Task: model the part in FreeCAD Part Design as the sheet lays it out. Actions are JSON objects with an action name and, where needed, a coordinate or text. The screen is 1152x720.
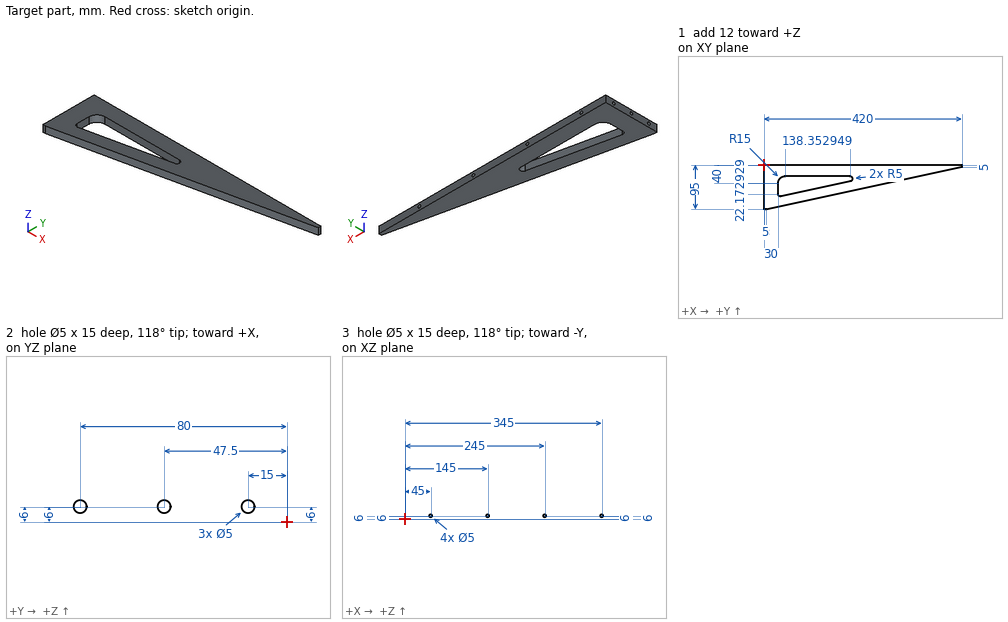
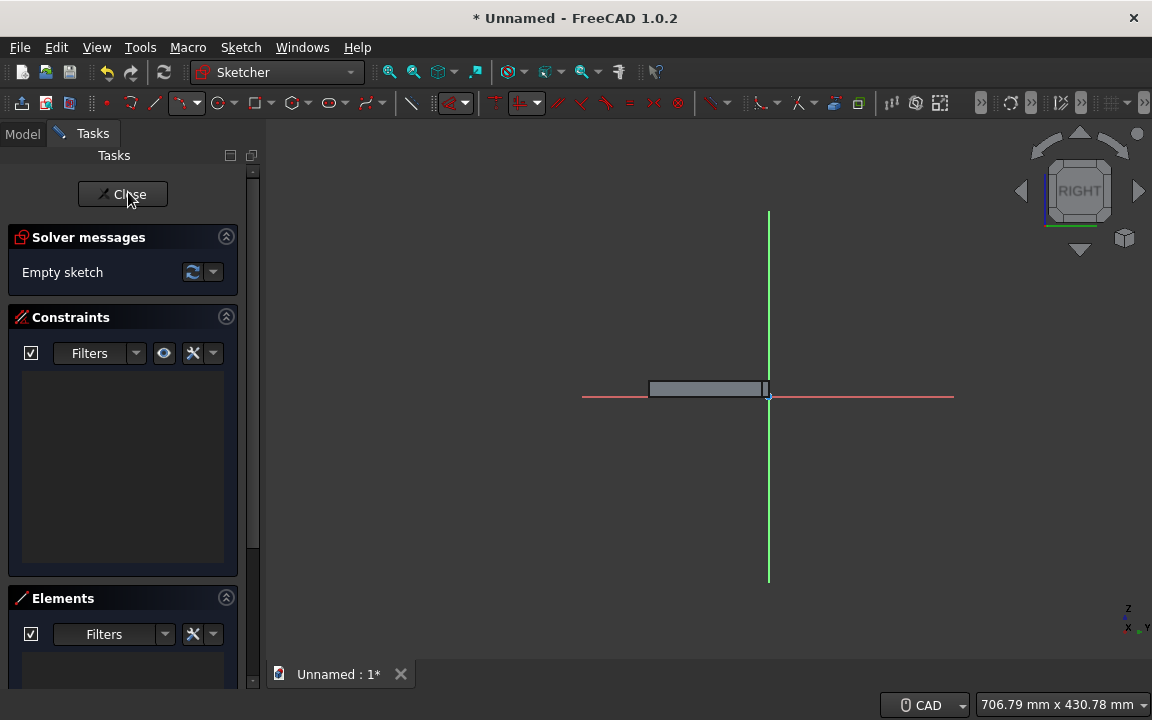
{"action": "left_click", "coordinate": [70, 104]}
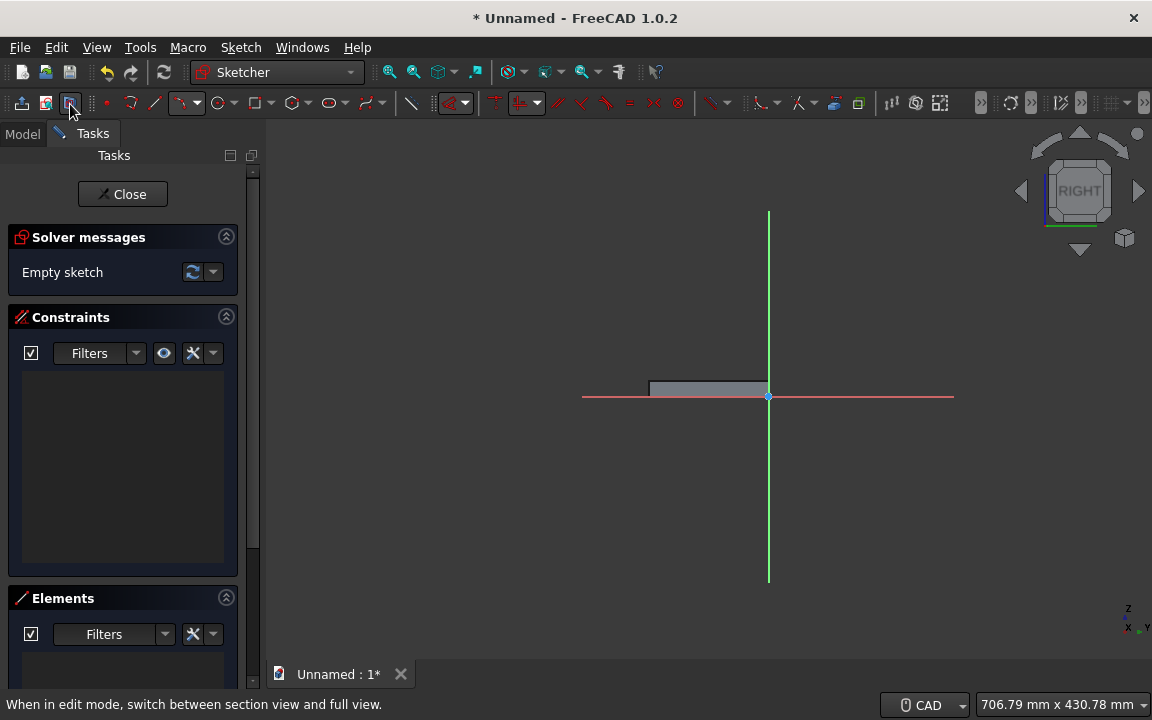
{"action": "scroll", "coordinate": [736, 392], "scroll_direction": "up", "scroll_amount": 8}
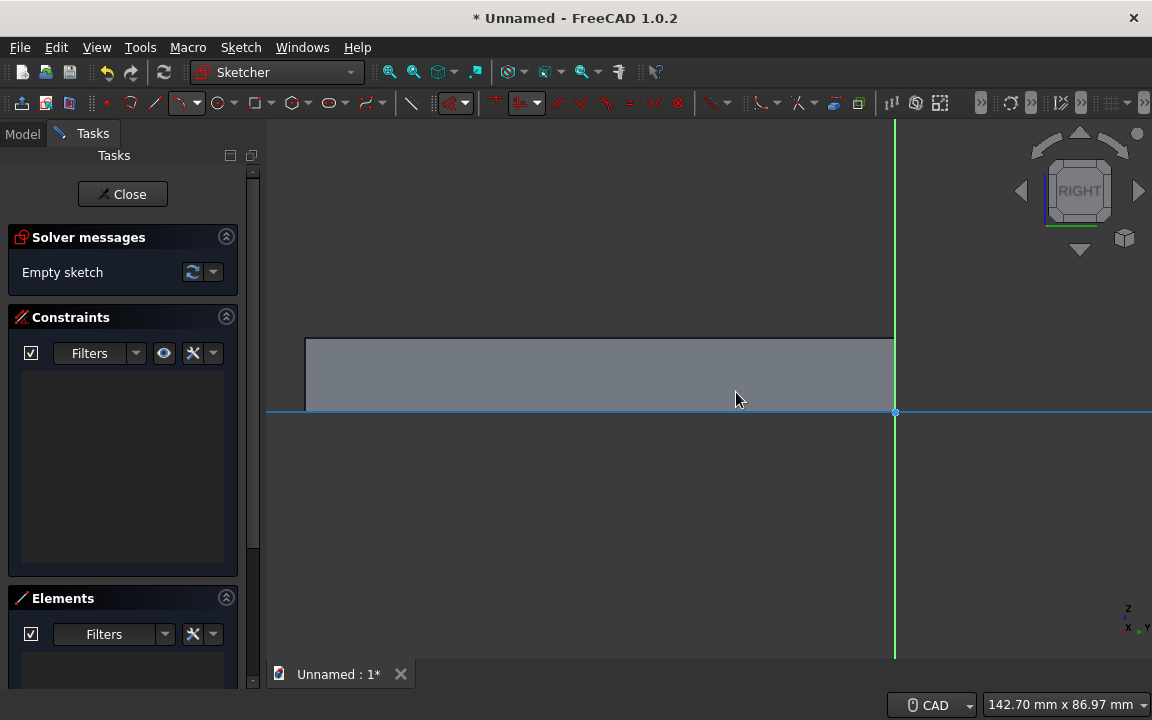
{"action": "left_click", "coordinate": [218, 104]}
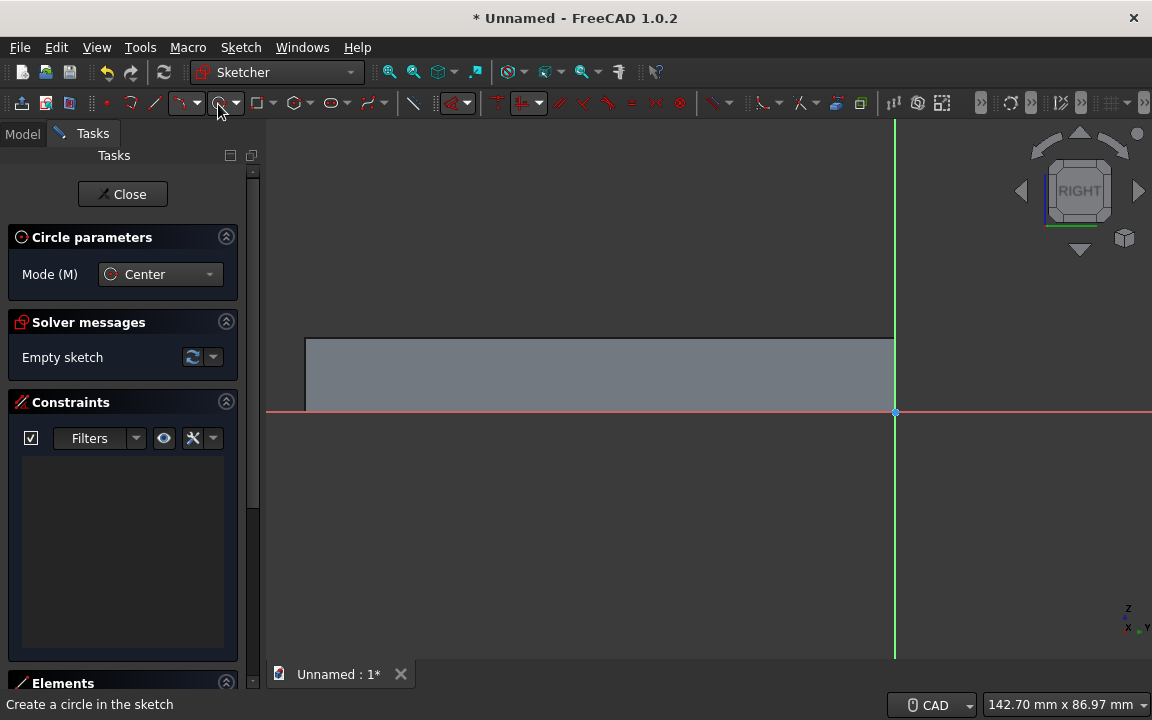
{"action": "scroll", "coordinate": [802, 375], "scroll_direction": "up", "scroll_amount": 2}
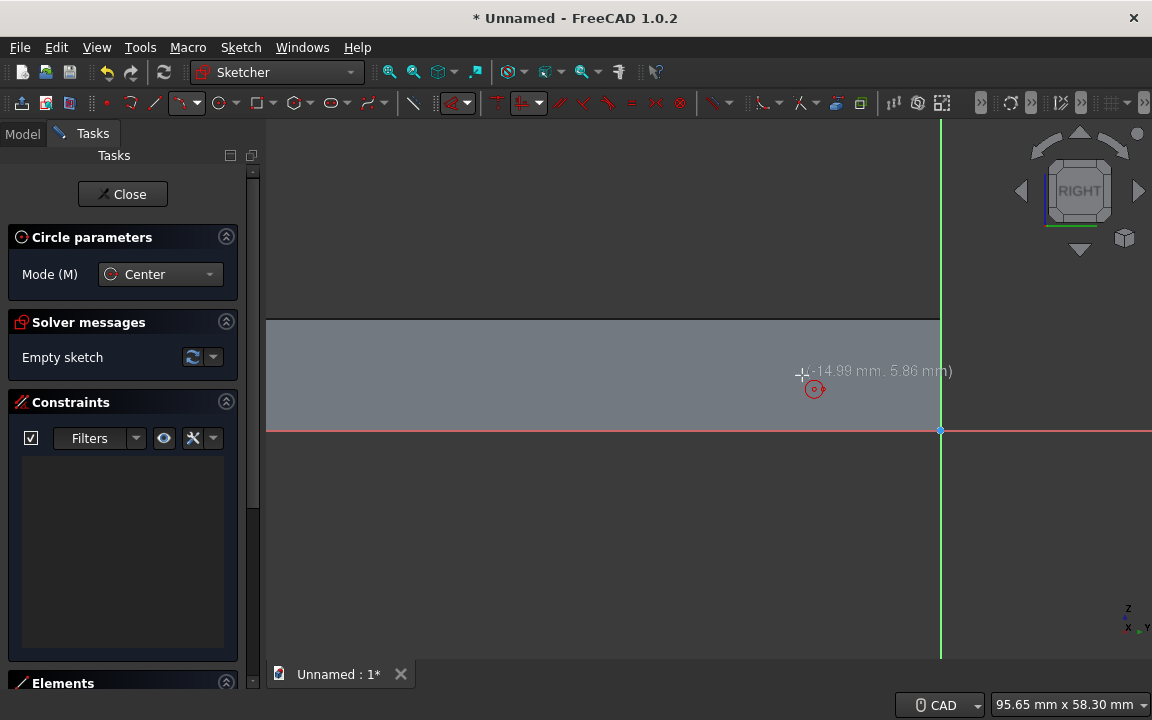
{"action": "left_click", "coordinate": [802, 375]}
{"action": "mouse_move", "coordinate": [818, 359]}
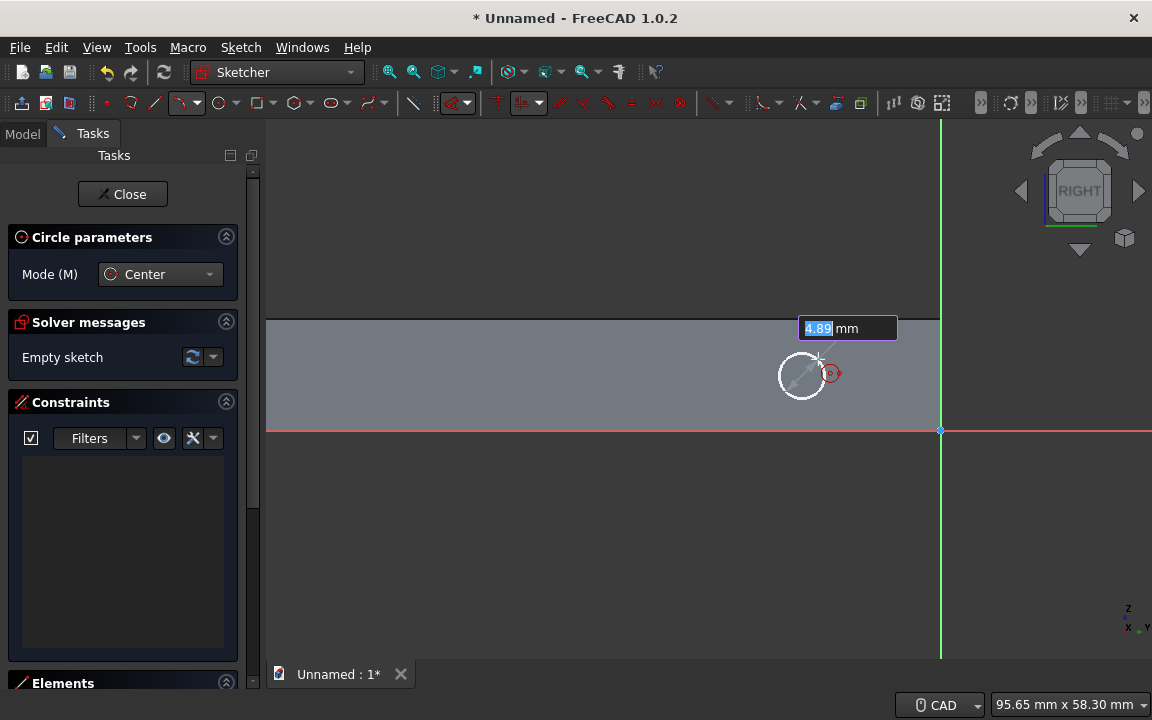
{"action": "type", "text": "5"}
{"action": "key", "text": "Return"}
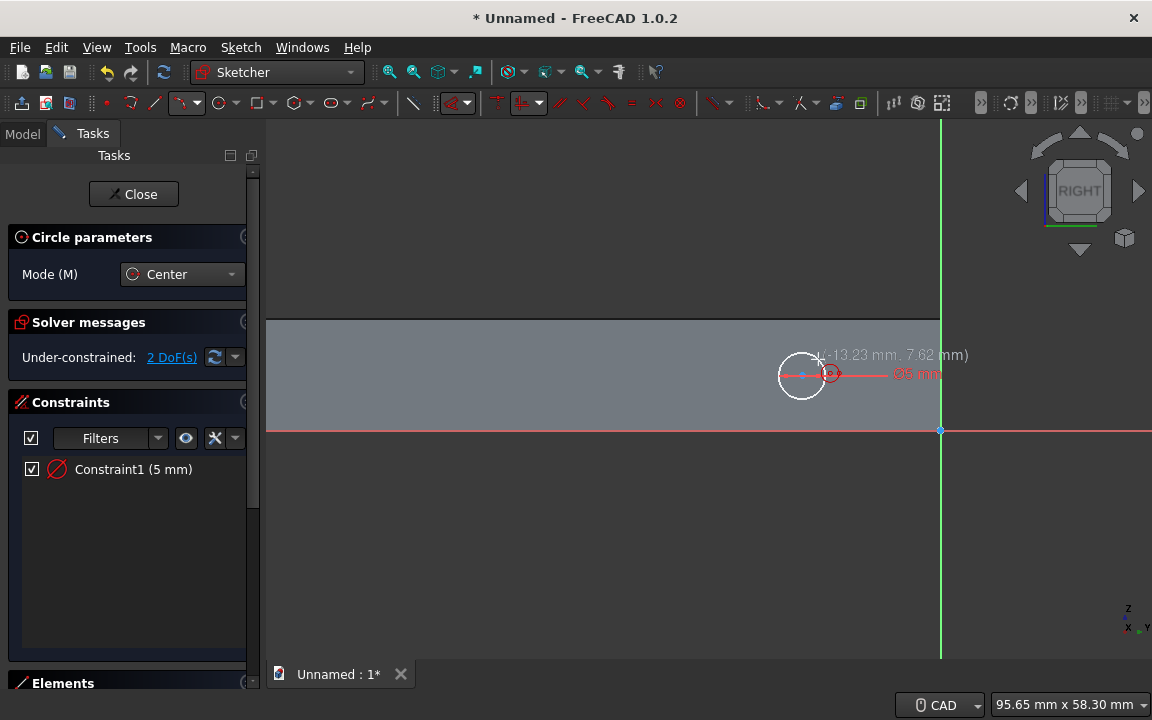
{"action": "left_click", "coordinate": [501, 375]}
{"action": "mouse_move", "coordinate": [517, 359]}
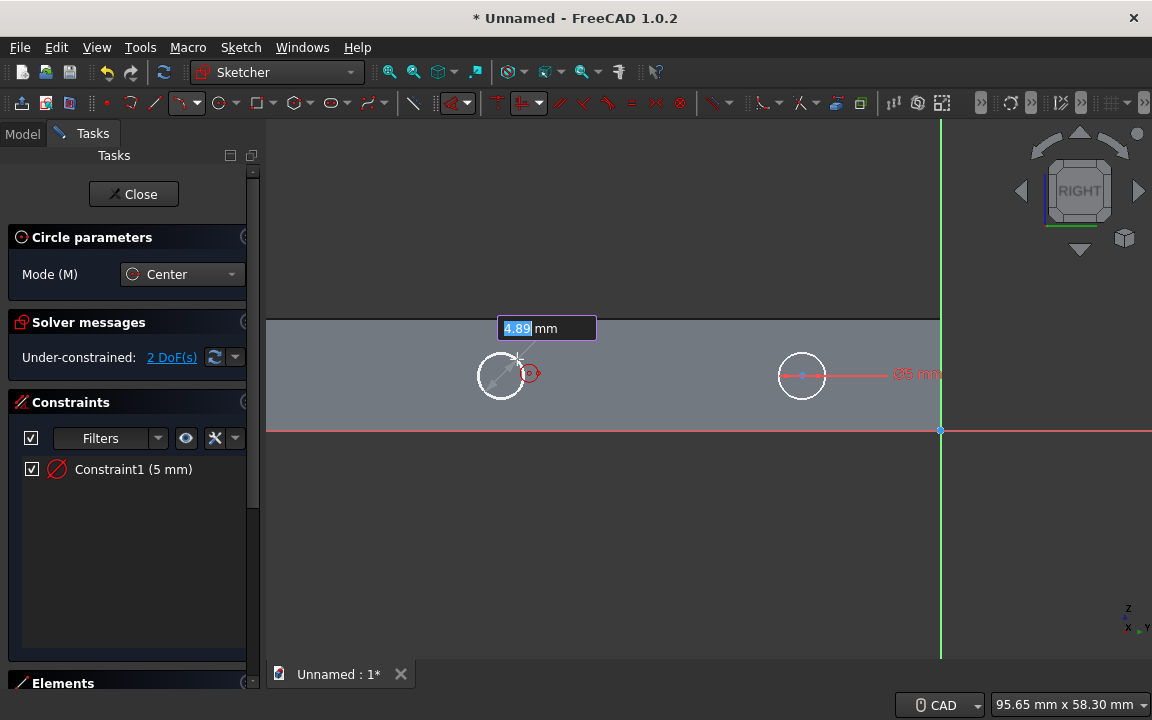
{"action": "type", "text": "5"}
{"action": "key", "text": "Return"}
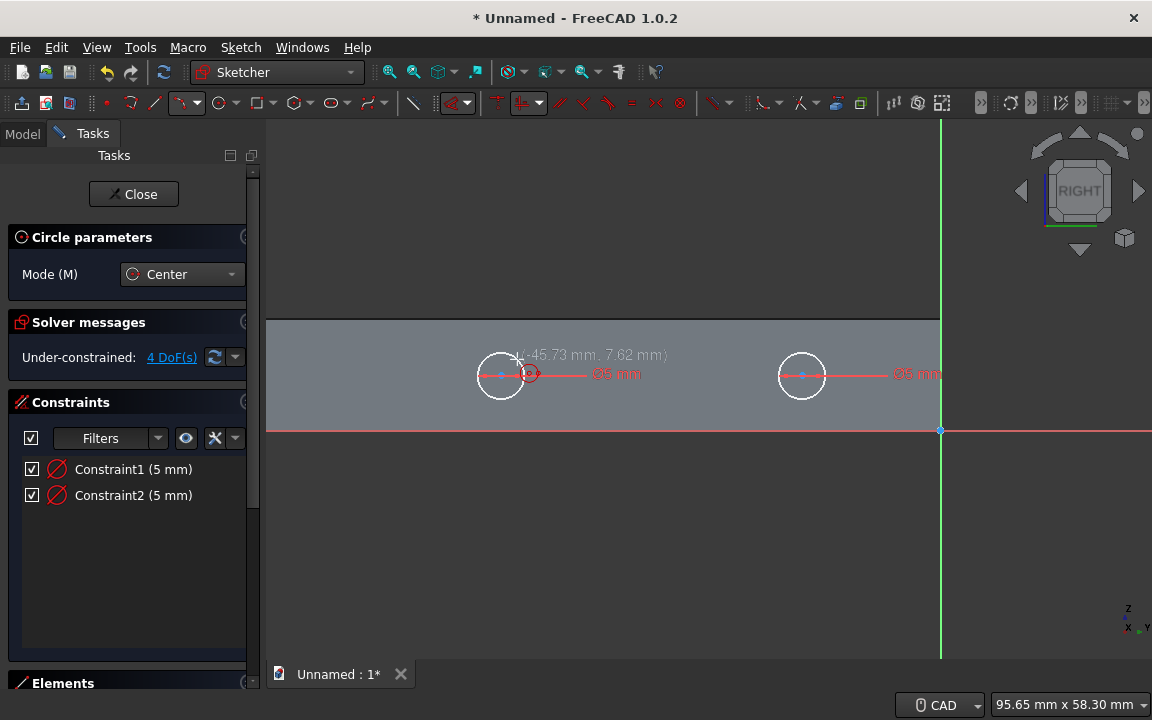
{"action": "scroll", "coordinate": [807, 385], "scroll_direction": "down", "scroll_amount": 2}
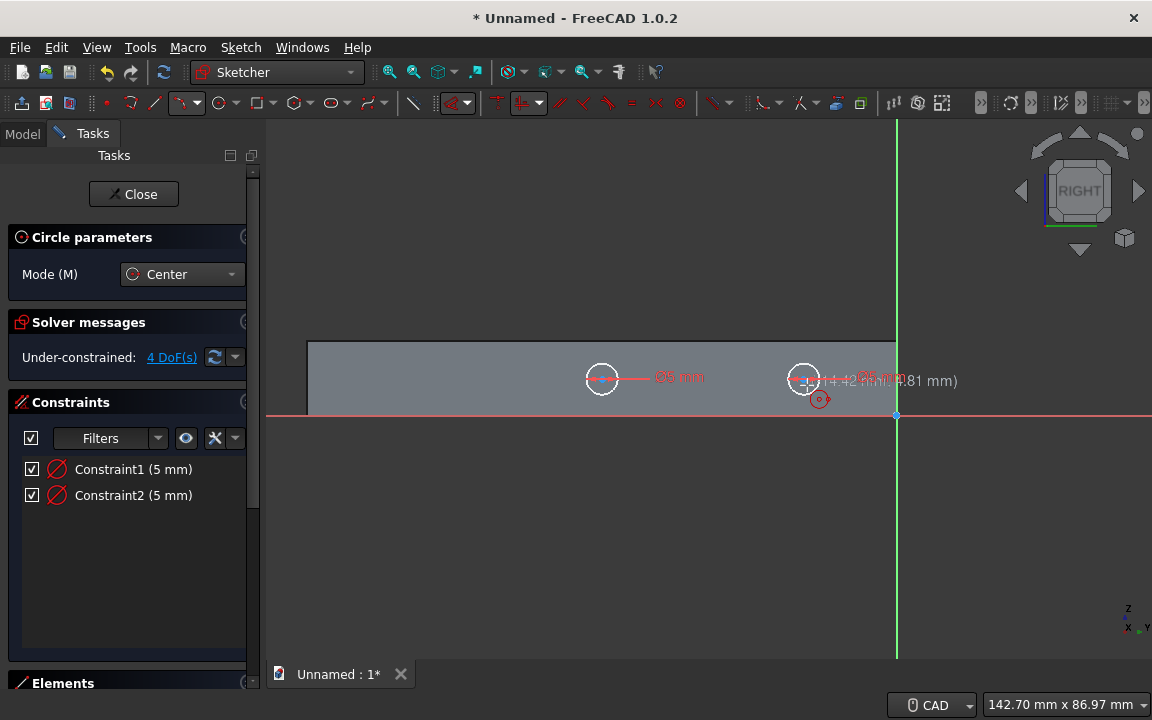
{"action": "scroll", "coordinate": [400, 378], "scroll_direction": "up", "scroll_amount": 2}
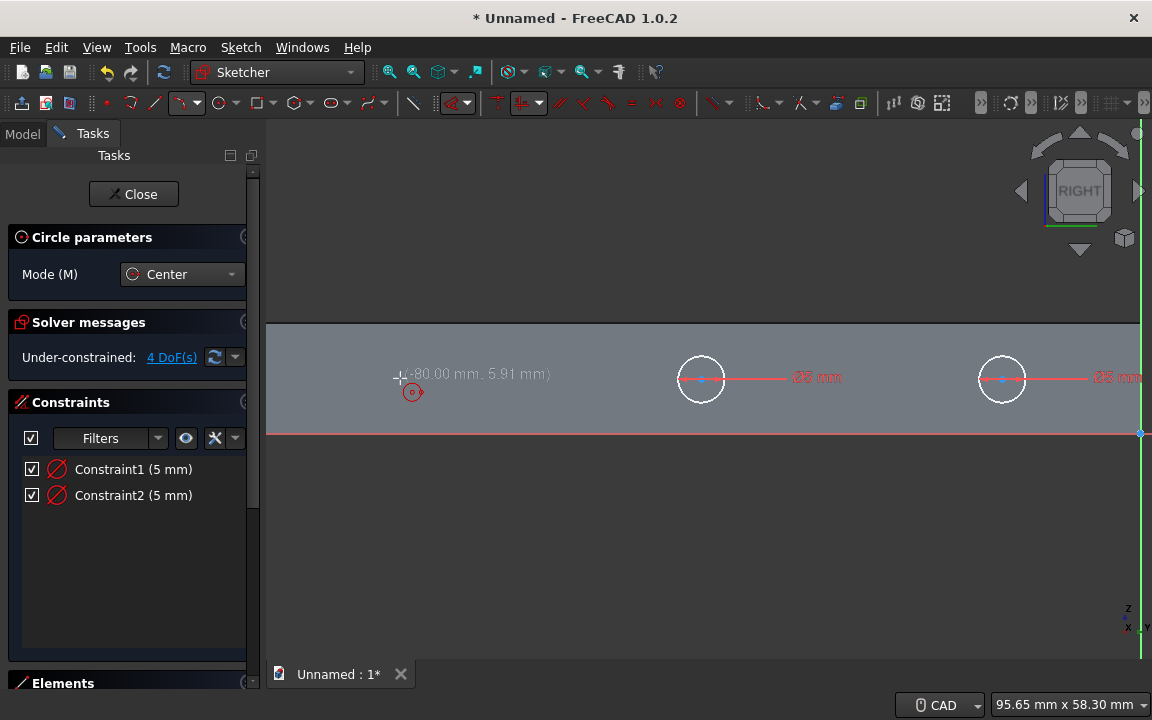
{"action": "left_click", "coordinate": [400, 378]}
{"action": "mouse_move", "coordinate": [416, 362]}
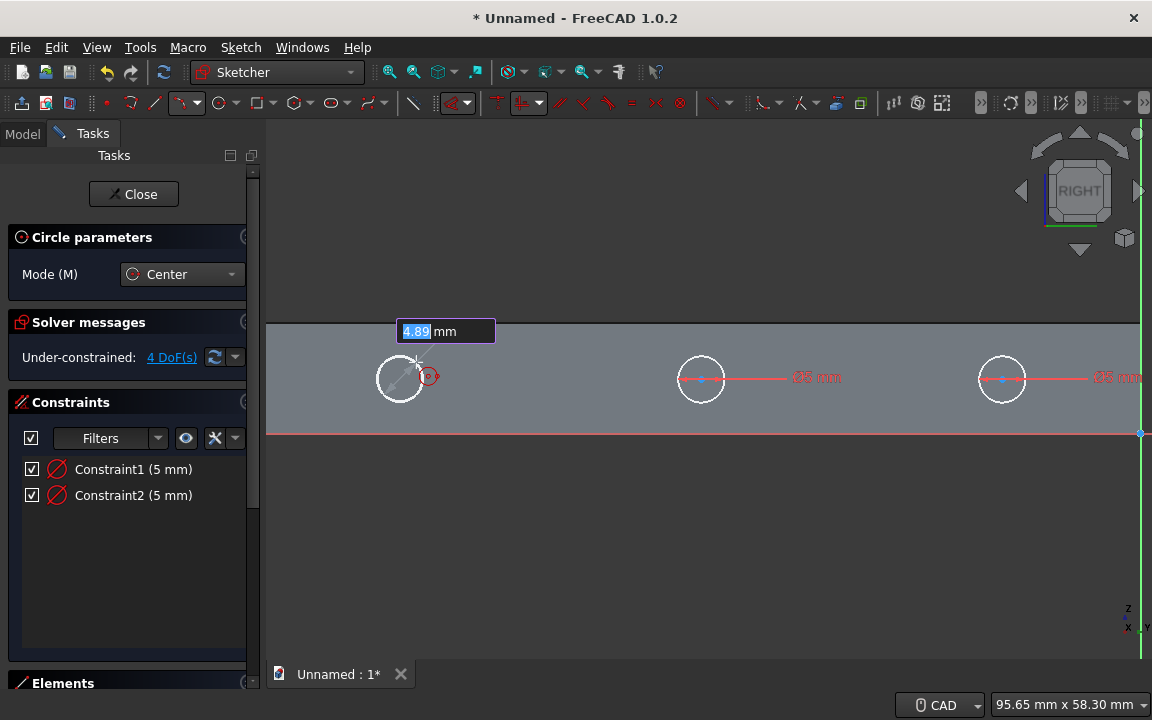
{"action": "type", "text": "5"}
{"action": "key", "text": "Return"}
{"action": "key", "text": "Escape"}